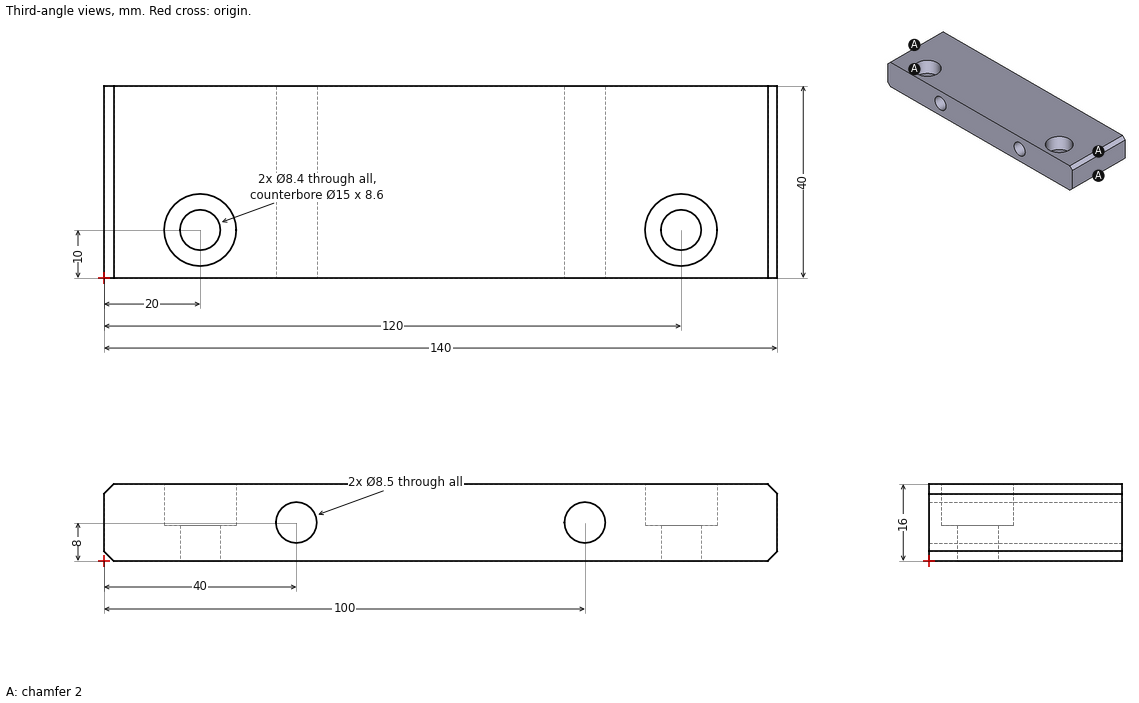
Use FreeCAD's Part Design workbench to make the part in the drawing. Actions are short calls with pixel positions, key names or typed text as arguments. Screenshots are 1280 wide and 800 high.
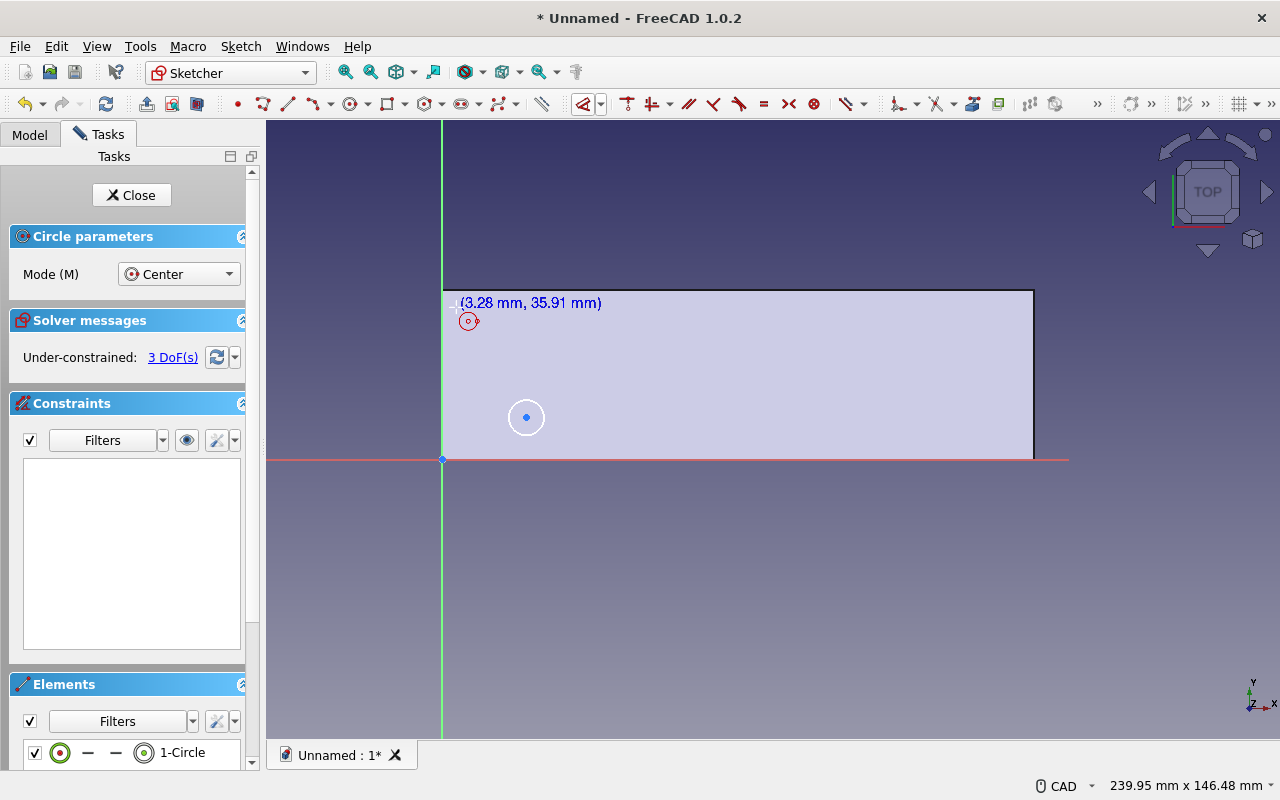
scroll(949, 417, up, 2)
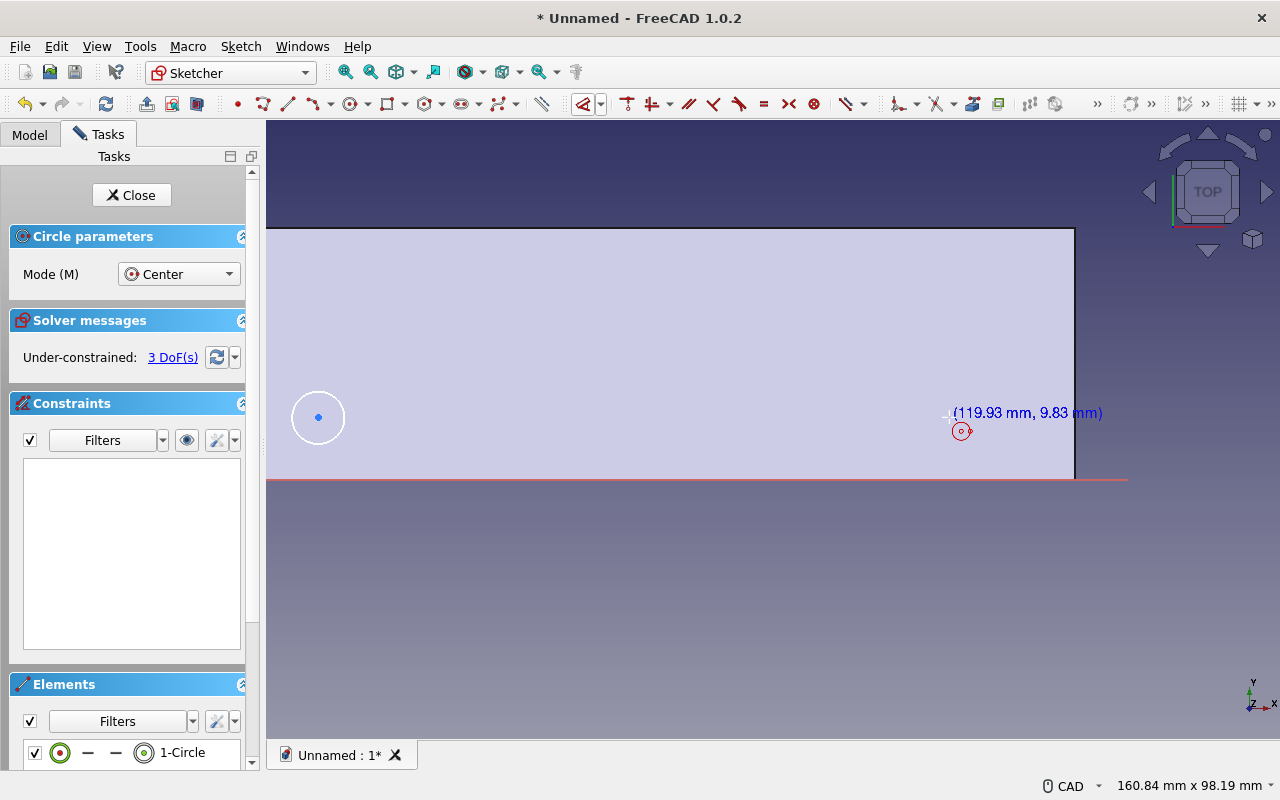
click(949, 417)
click(968, 398)
key(Escape)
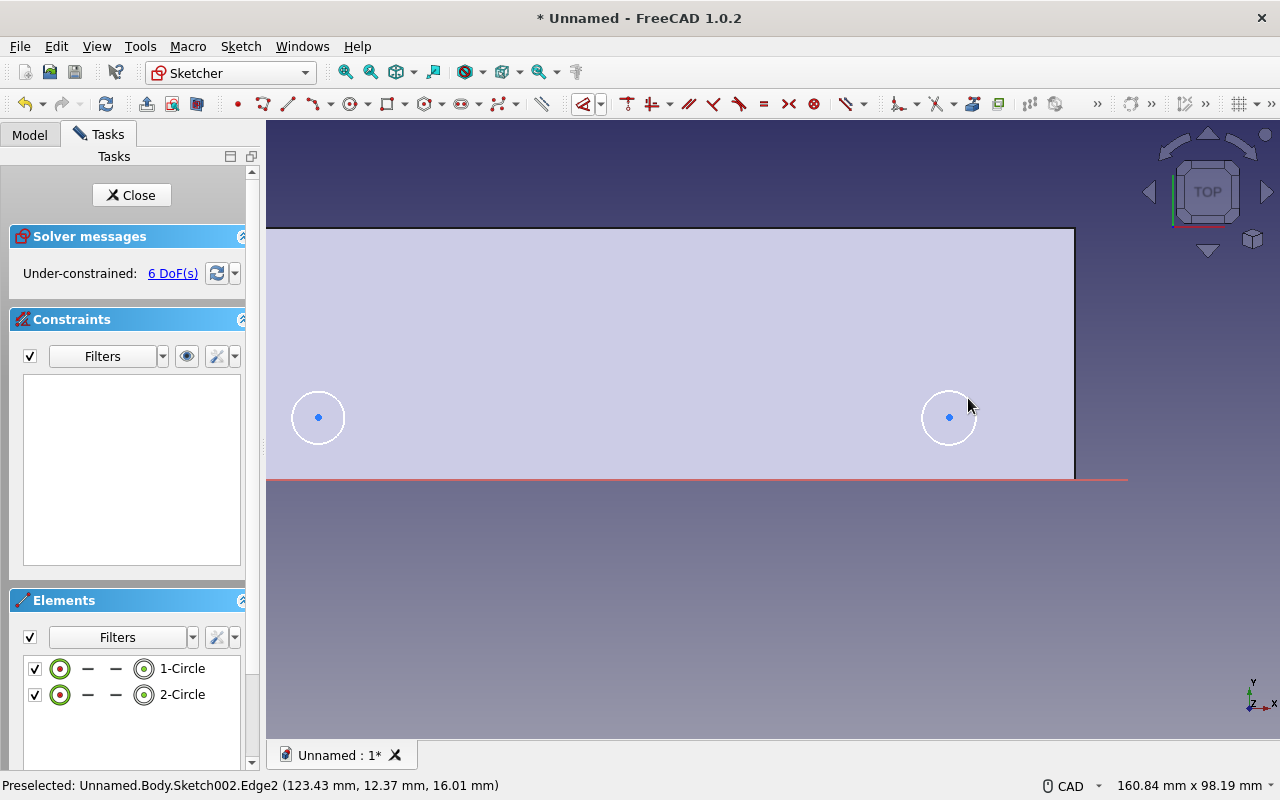
click(337, 399)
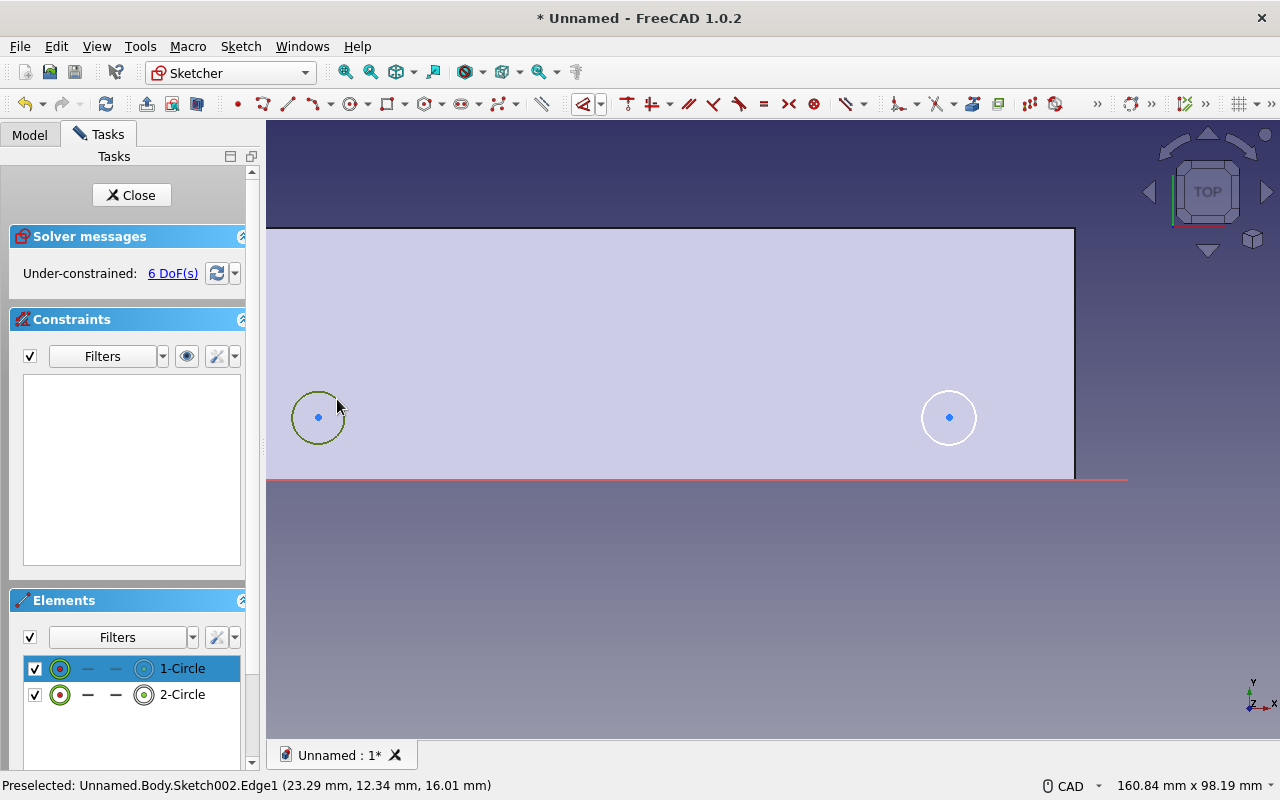
click(968, 399)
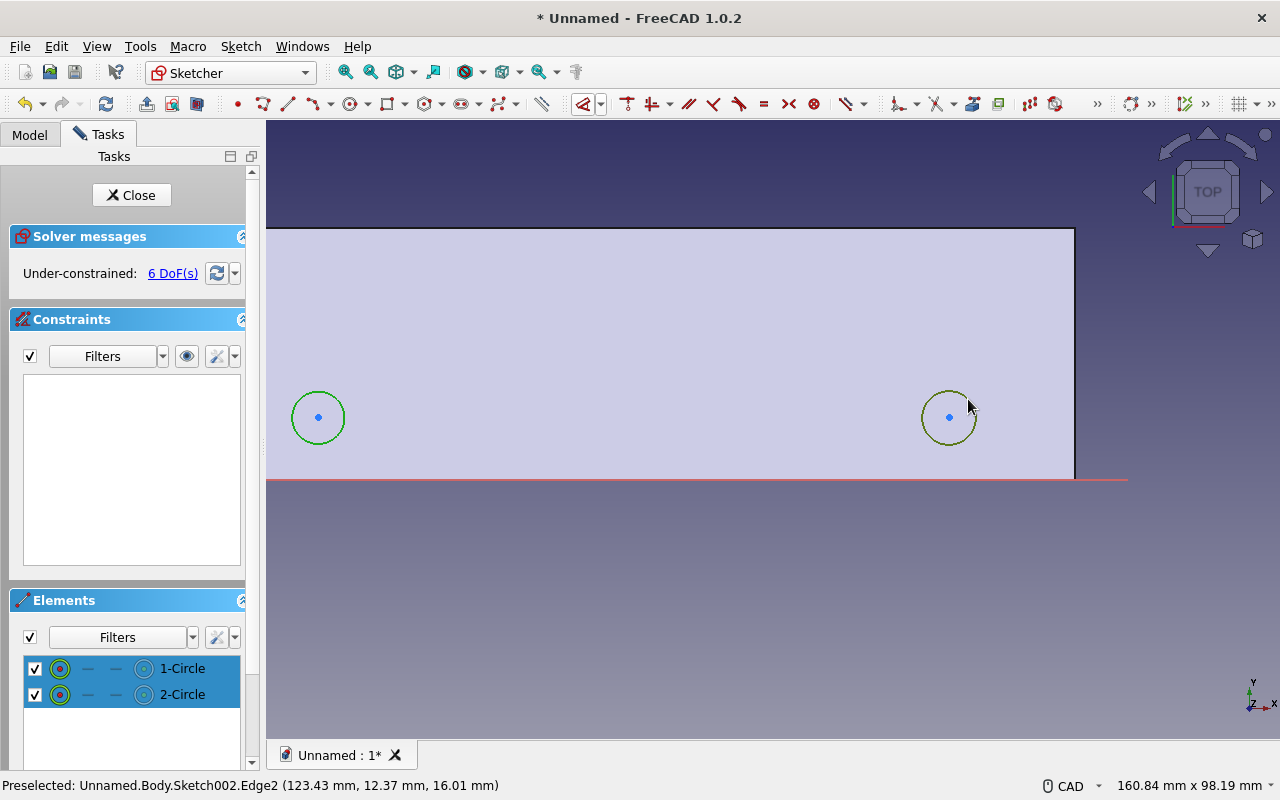
click(764, 104)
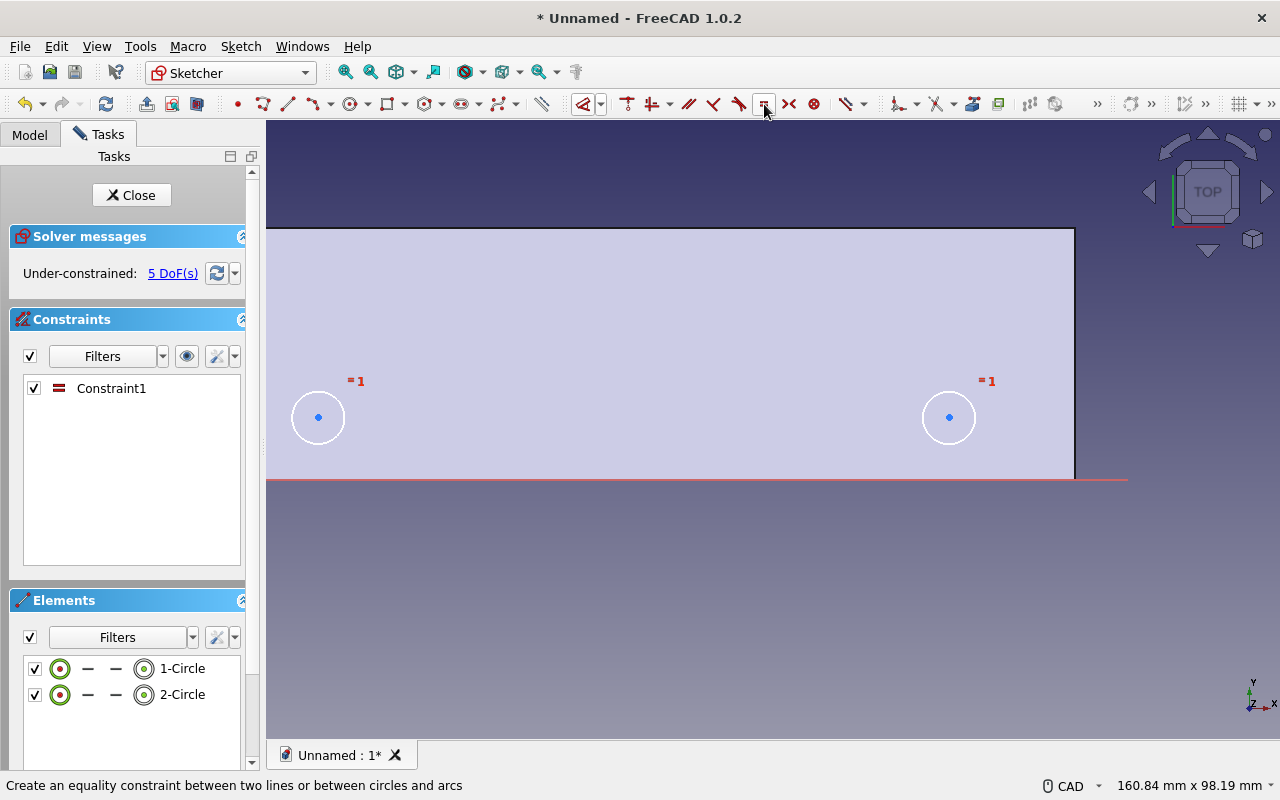
click(337, 399)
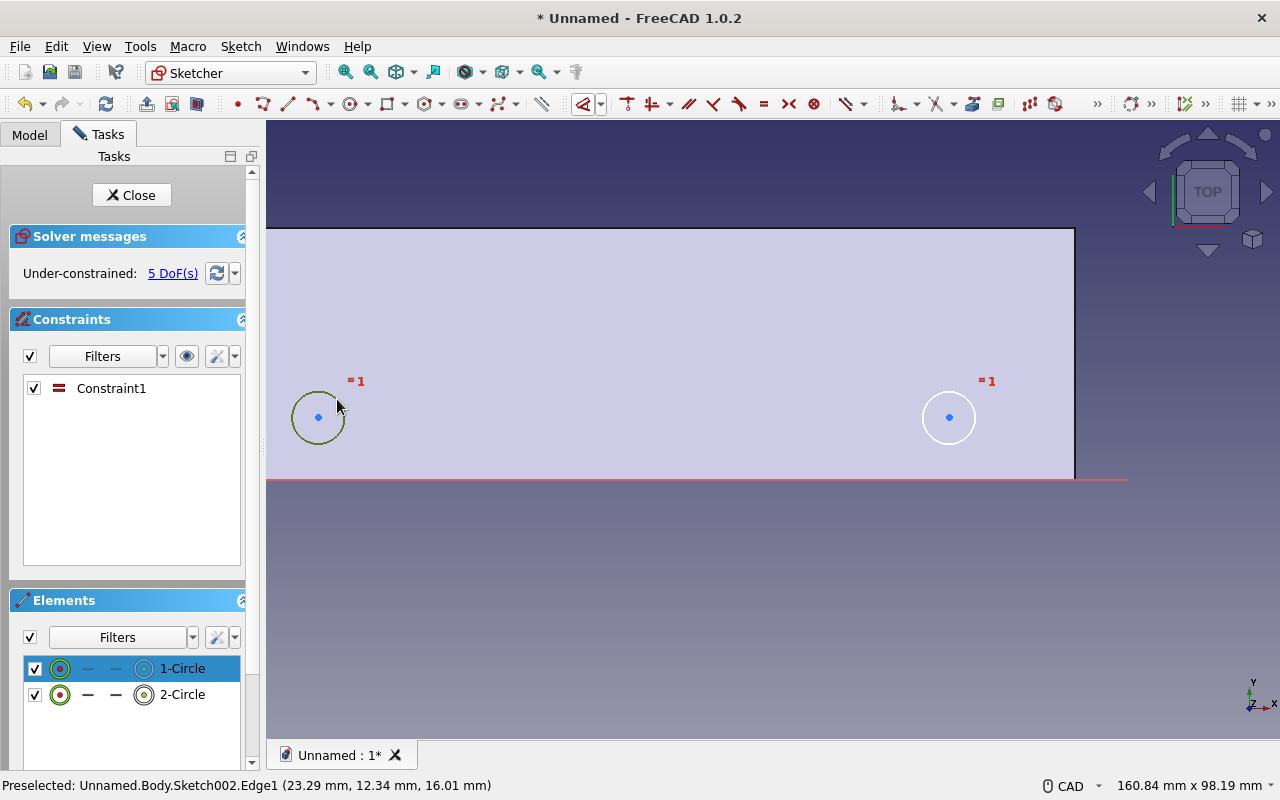
key(k)
key(o)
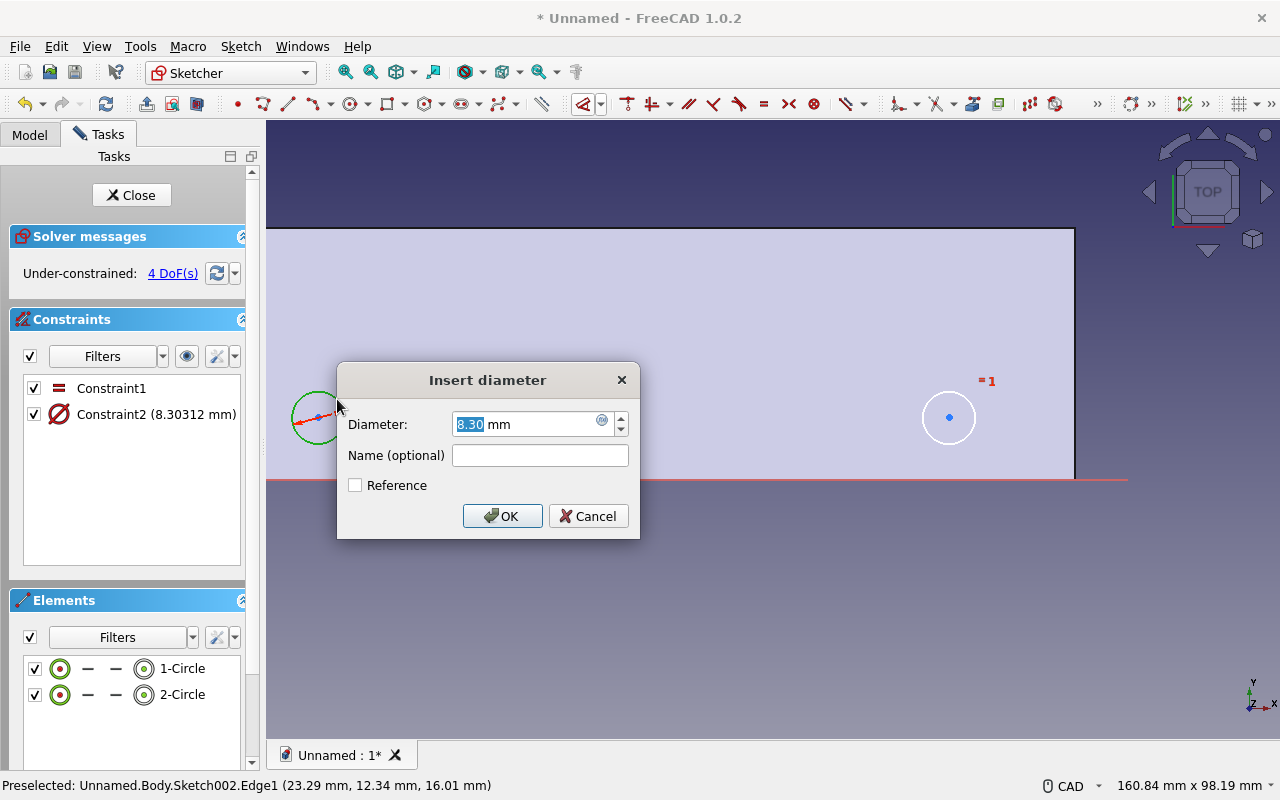
text(8.4)
key(Return)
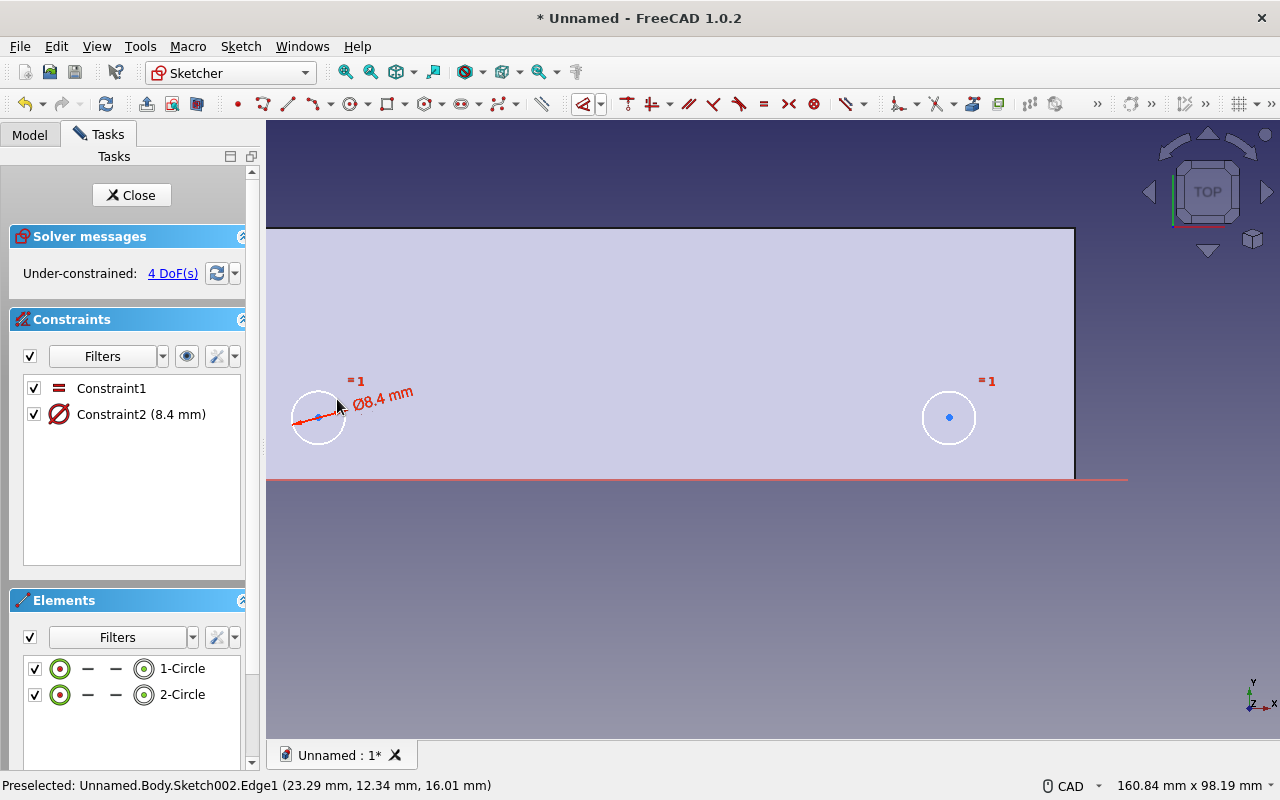
click(318, 418)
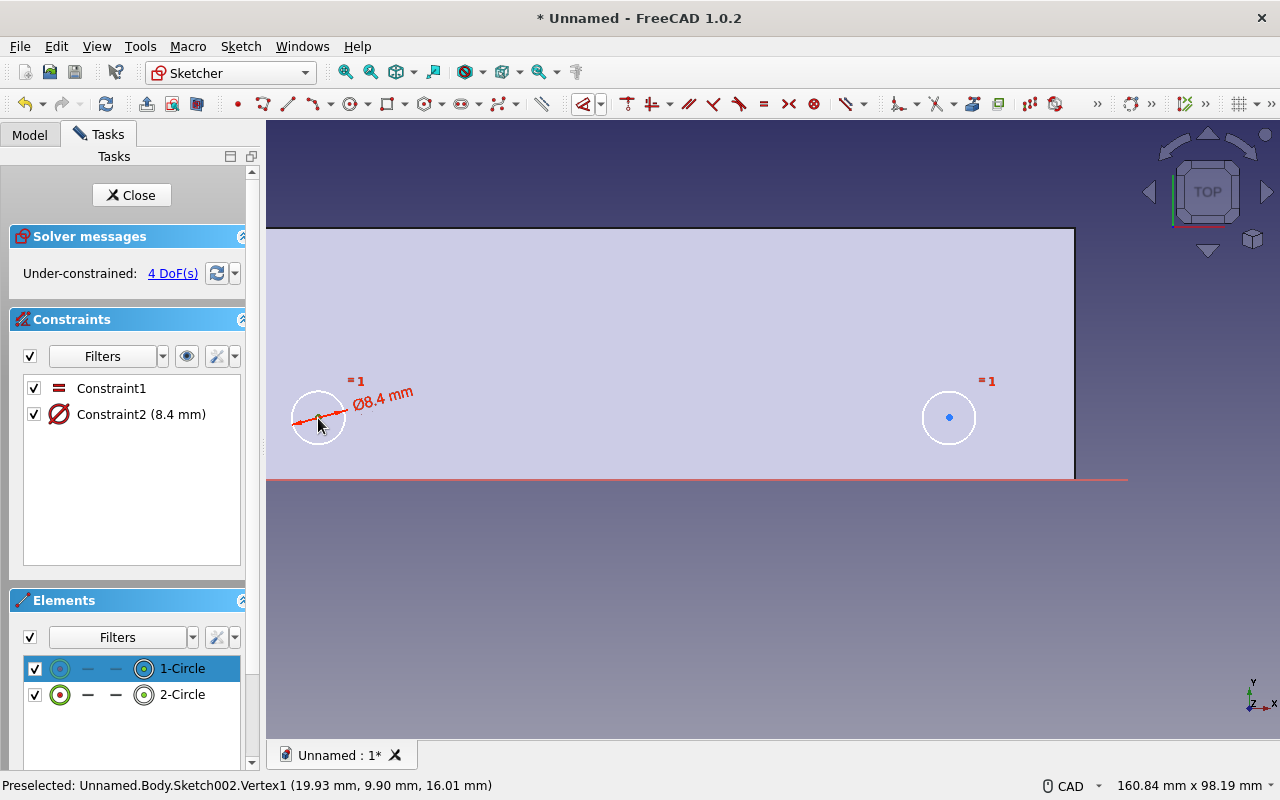
click(600, 104)